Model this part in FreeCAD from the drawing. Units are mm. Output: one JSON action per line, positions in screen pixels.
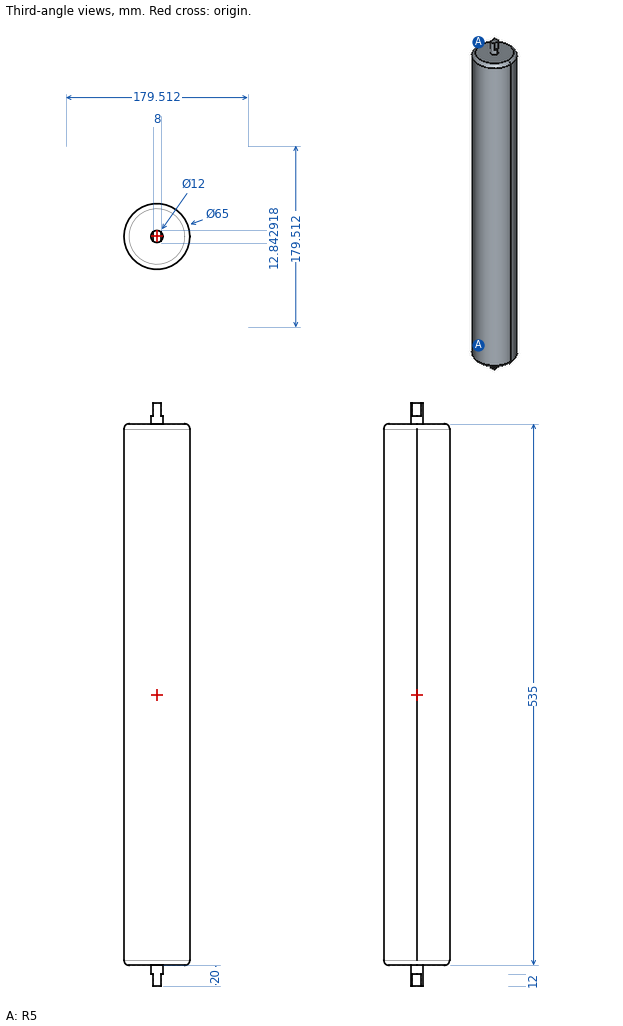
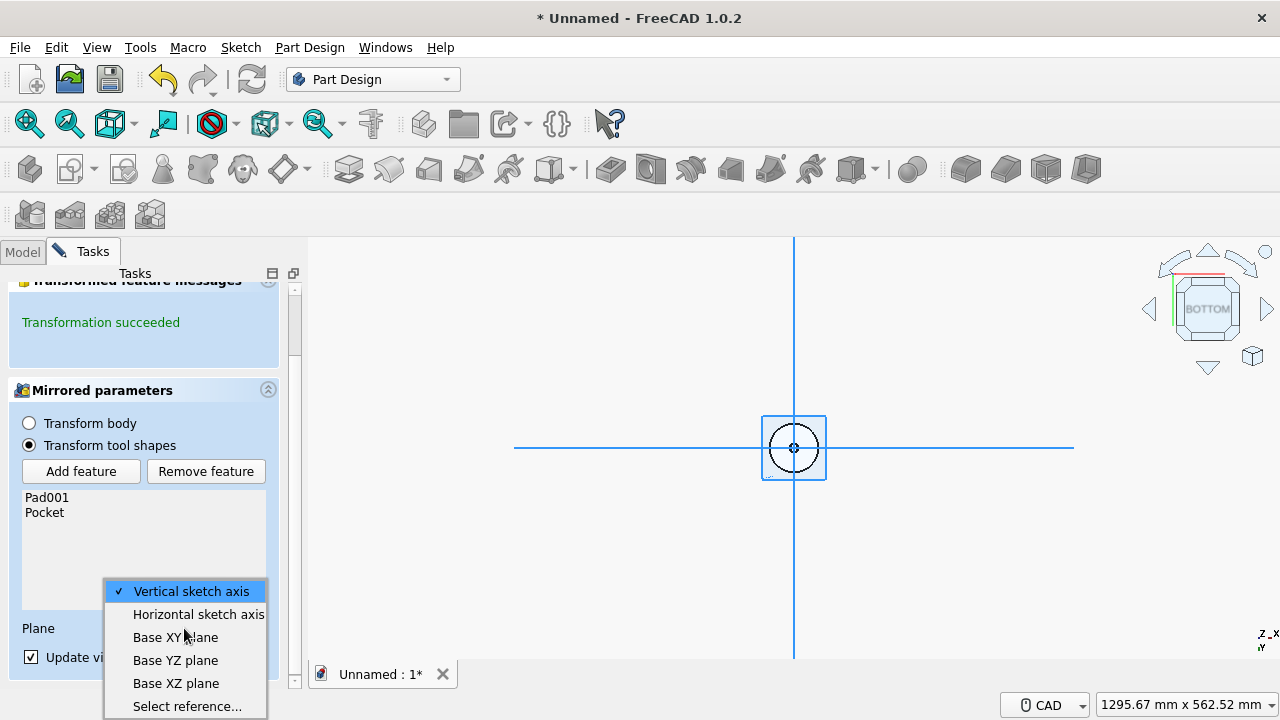
{"action": "left_click", "coordinate": [184, 638]}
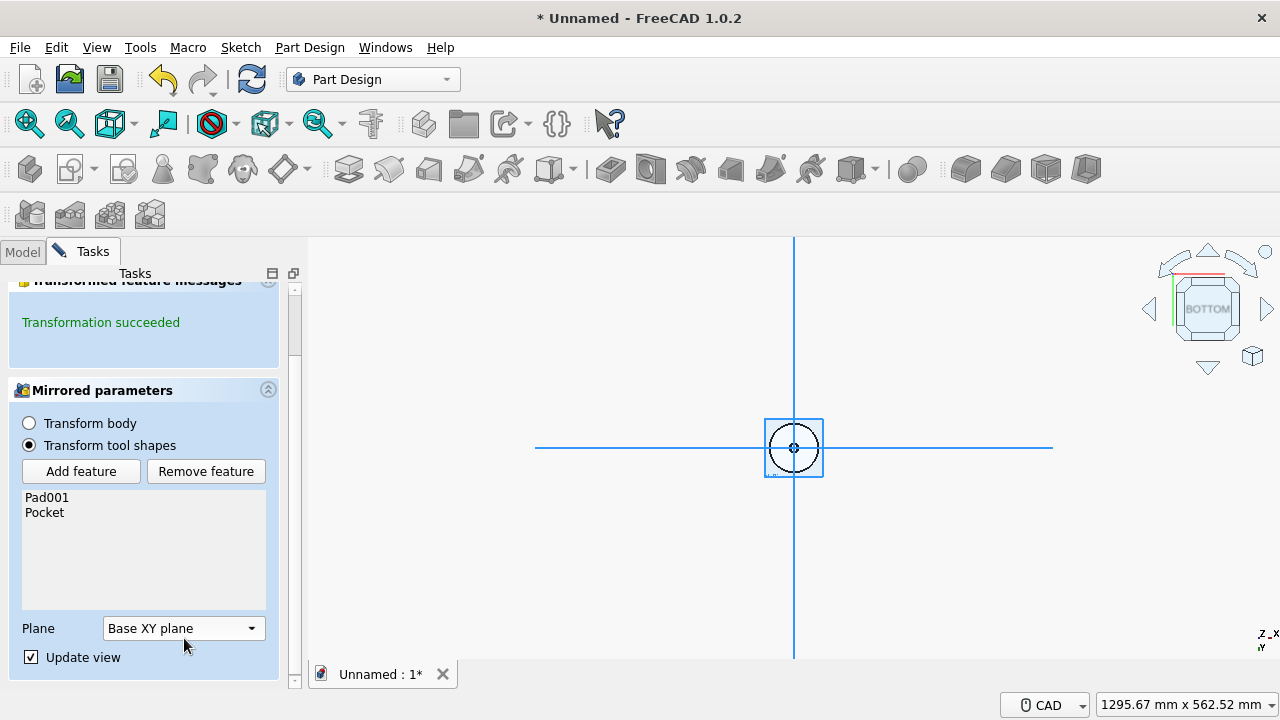
{"action": "scroll", "coordinate": [295, 486], "scroll_direction": "up", "scroll_amount": 2}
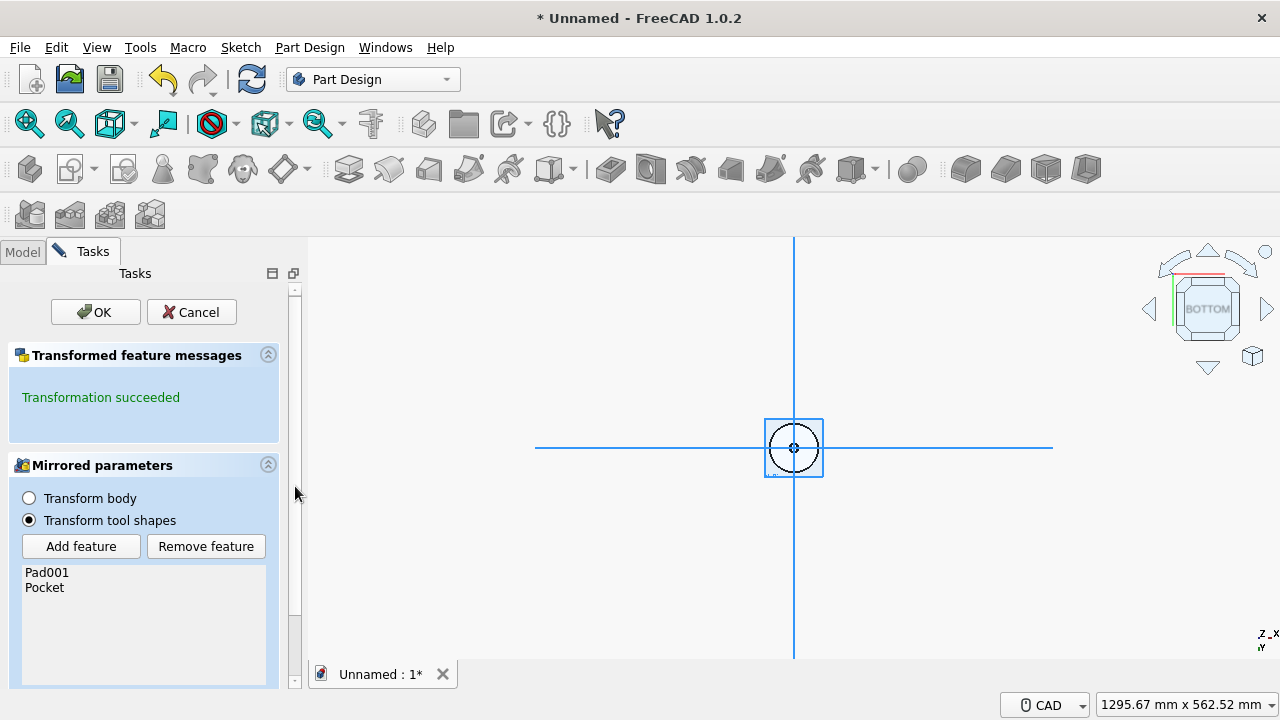
{"action": "left_click", "coordinate": [96, 312]}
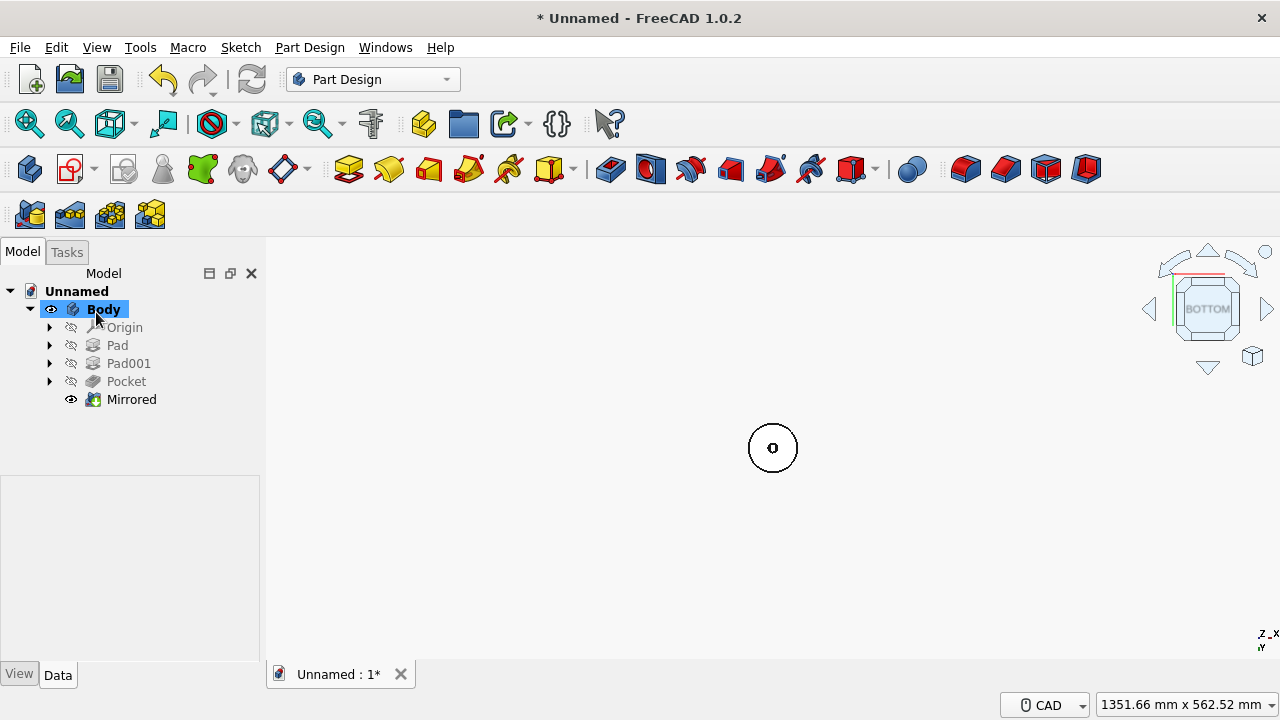
{"action": "left_click", "coordinate": [30, 124]}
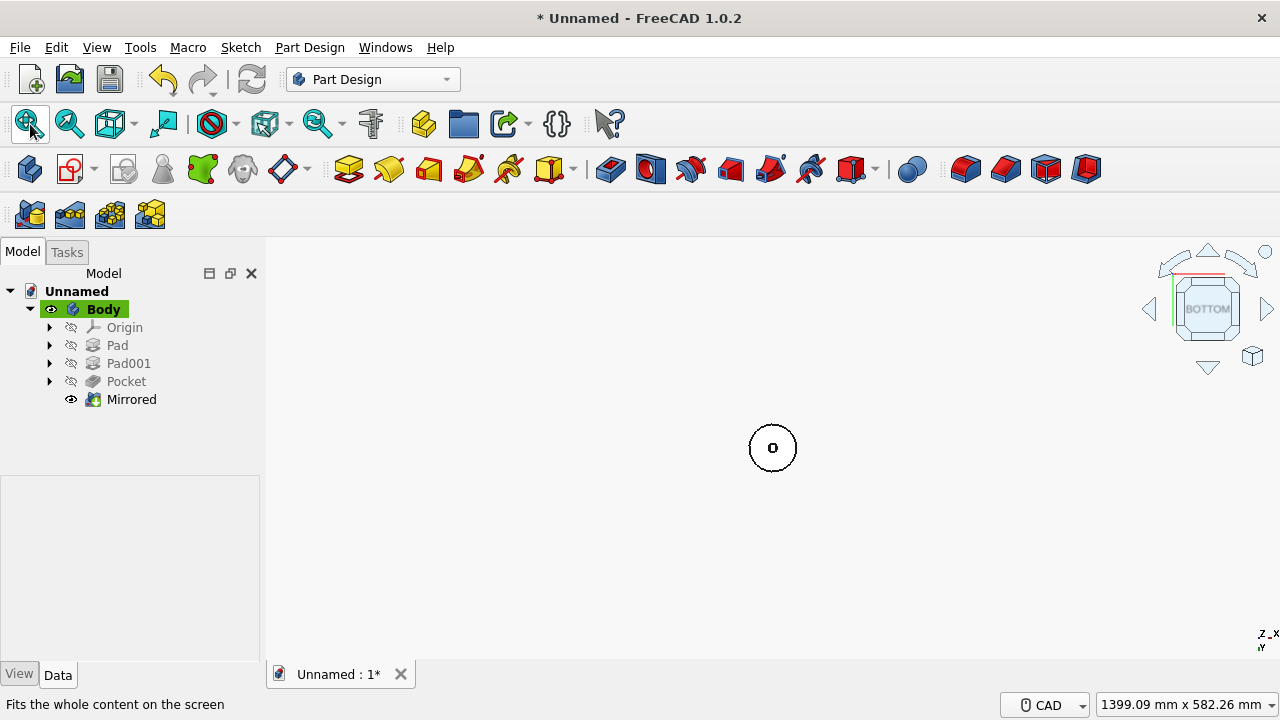
{"action": "left_click", "coordinate": [749, 447]}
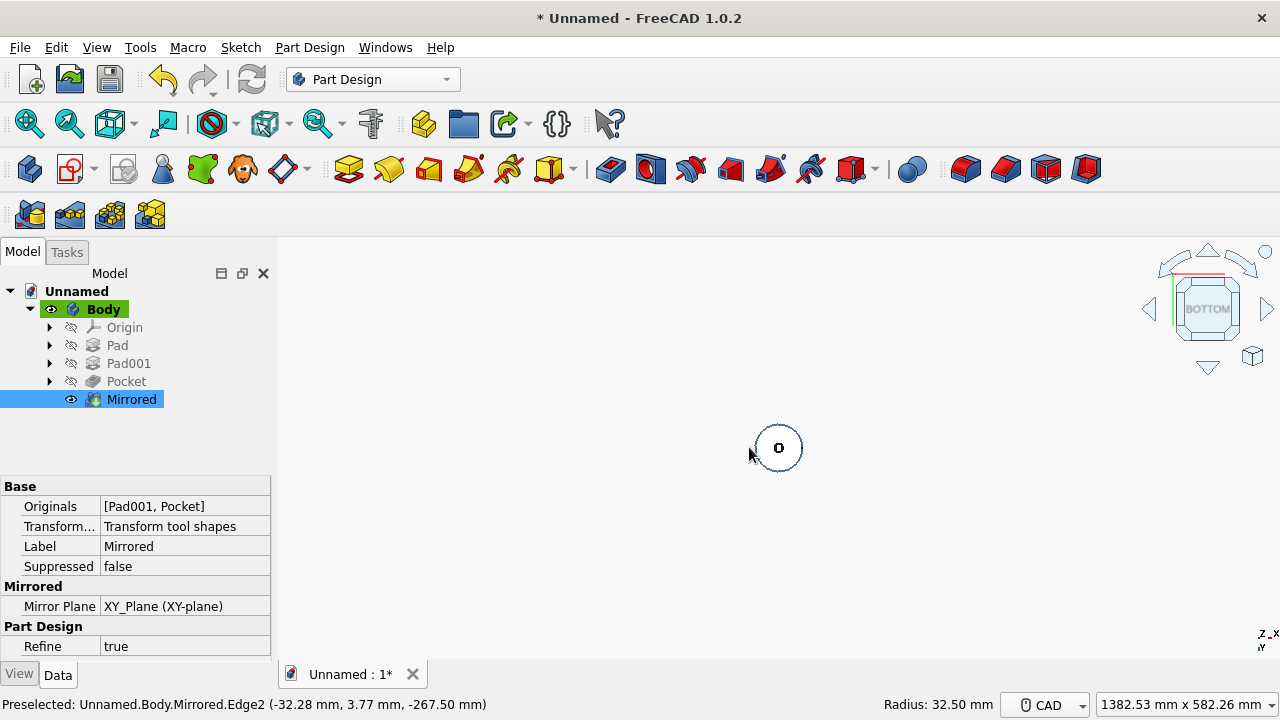
{"action": "key", "text": "0"}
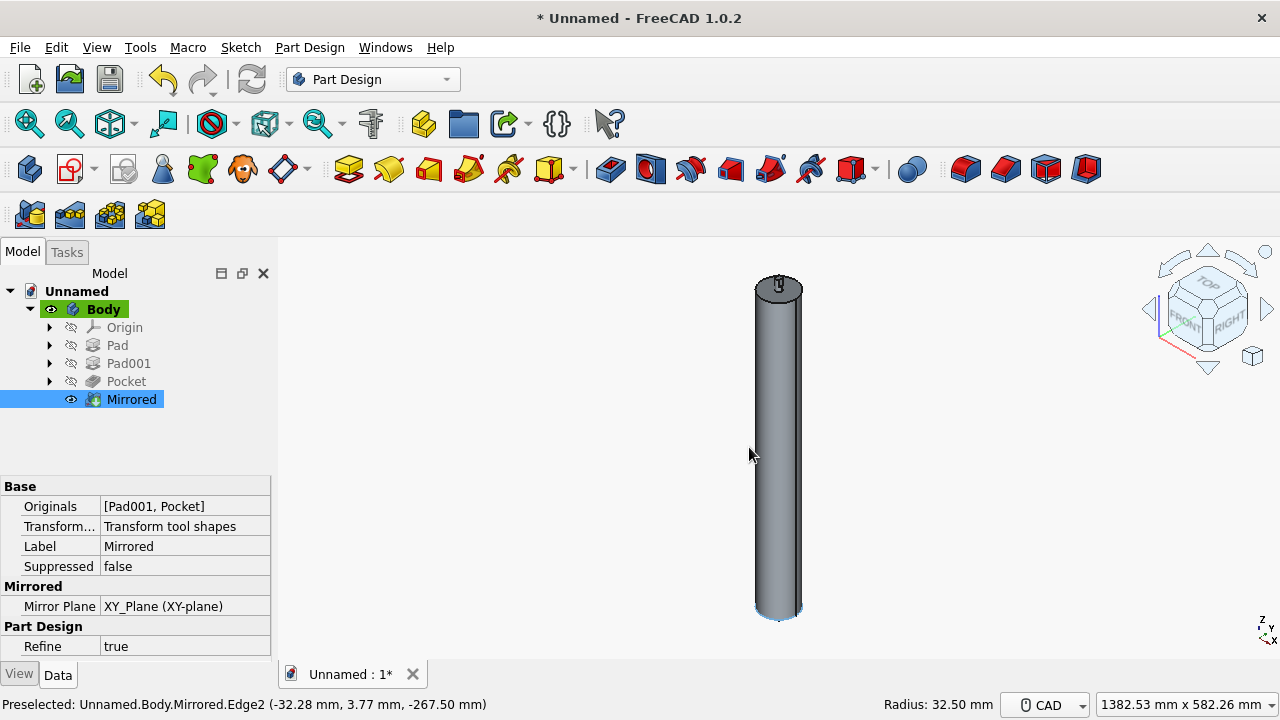
{"action": "left_click", "coordinate": [762, 279], "text": "ctrl"}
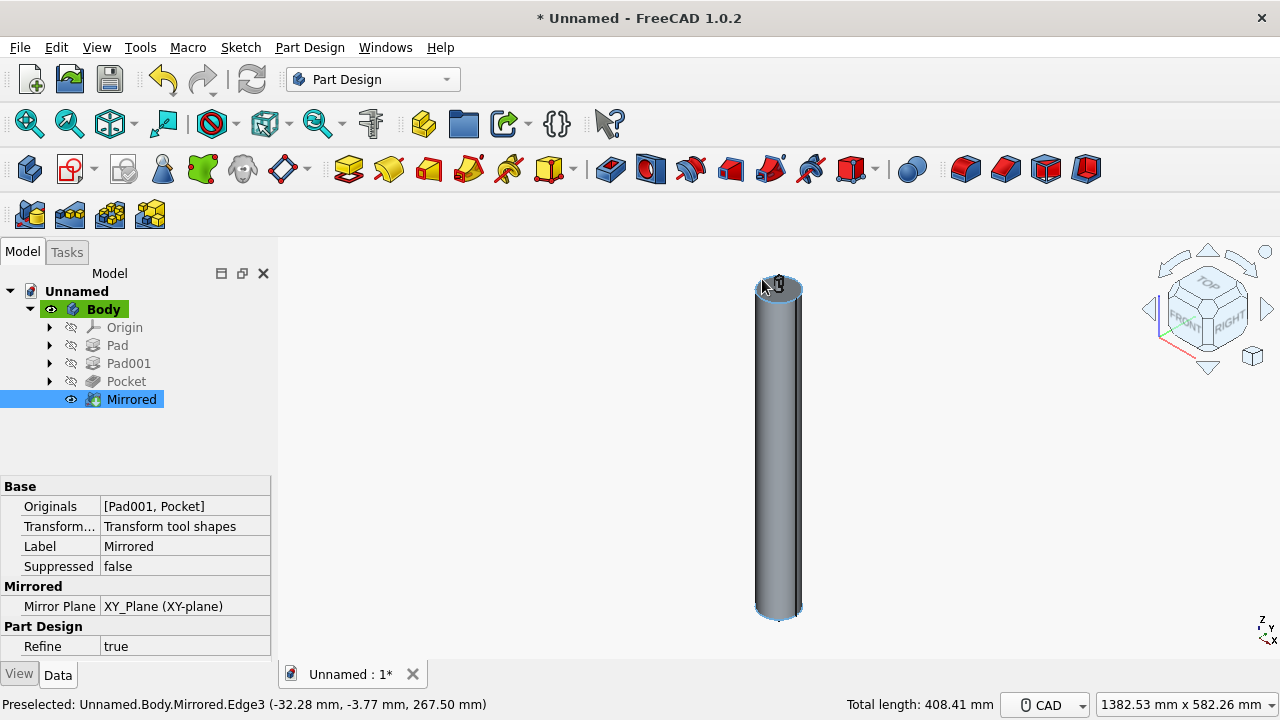
{"action": "left_click", "coordinate": [966, 170]}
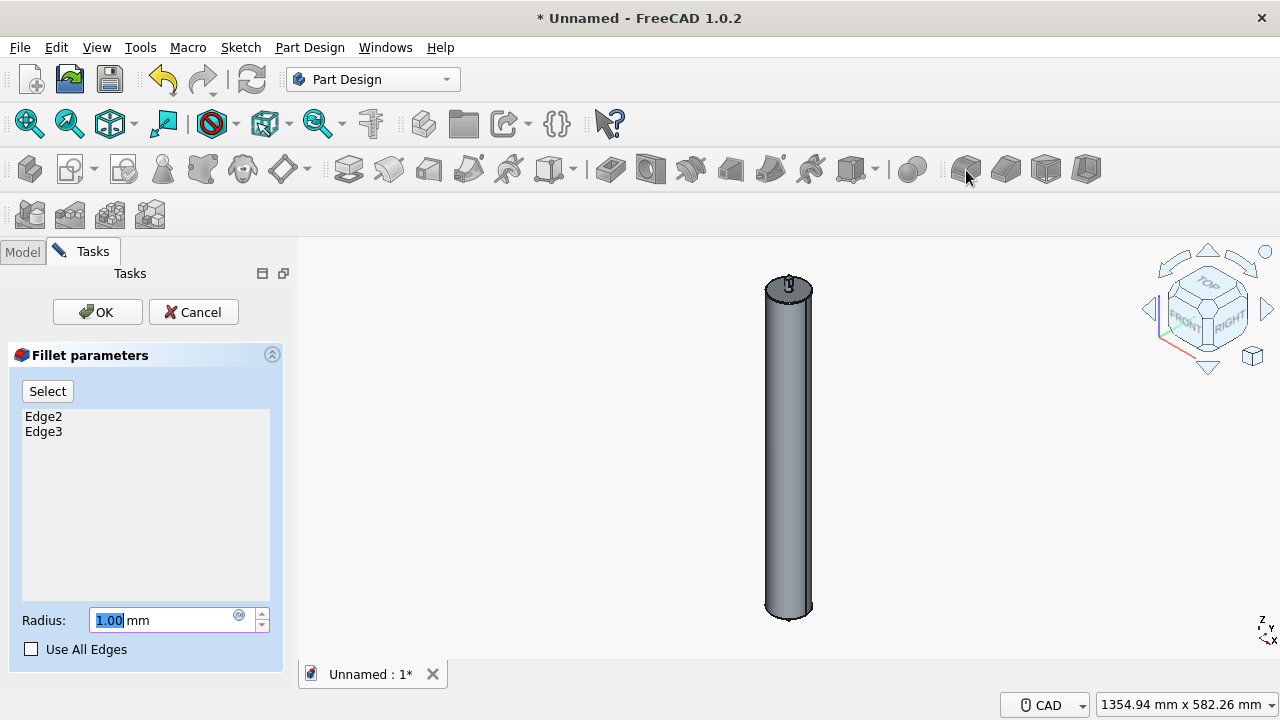
{"action": "type", "text": "5"}
{"action": "key", "text": "Tab"}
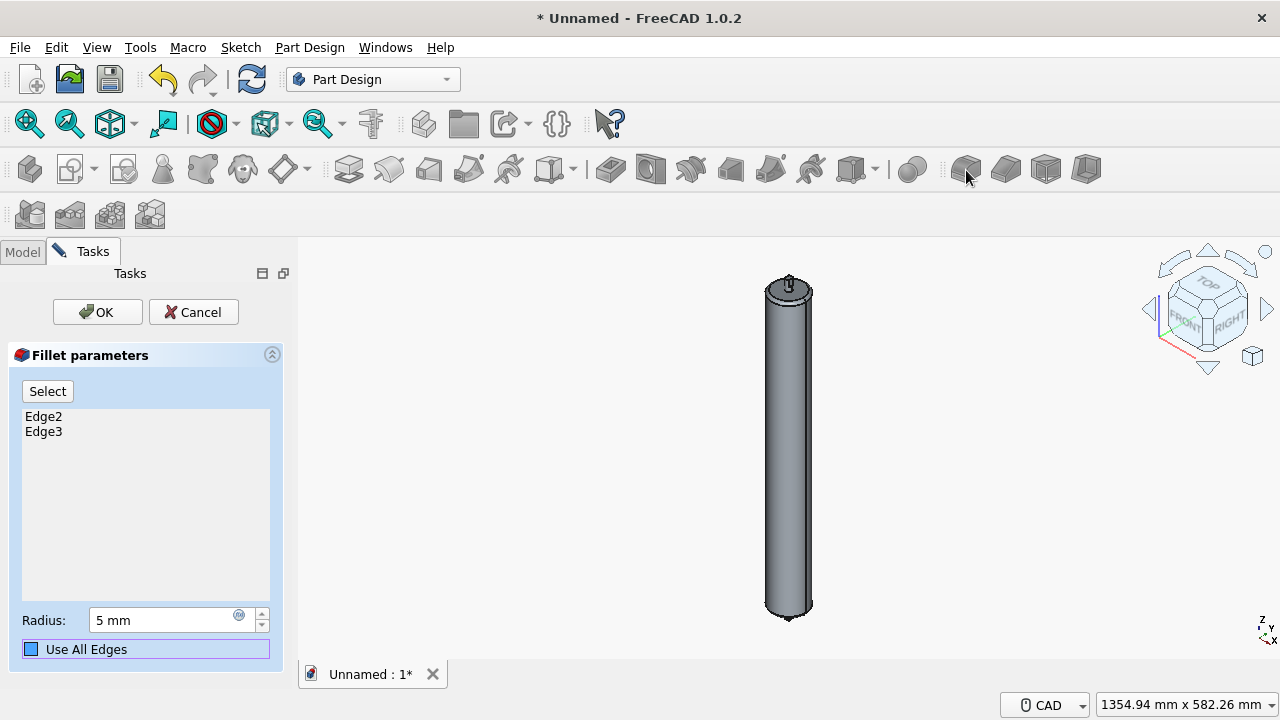
{"action": "left_click", "coordinate": [98, 312]}